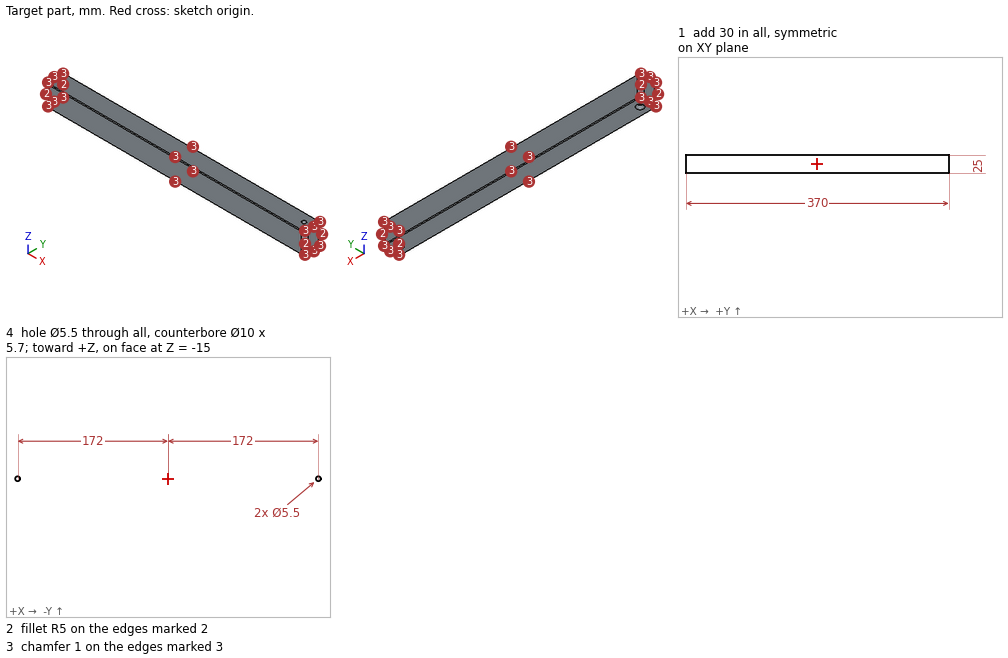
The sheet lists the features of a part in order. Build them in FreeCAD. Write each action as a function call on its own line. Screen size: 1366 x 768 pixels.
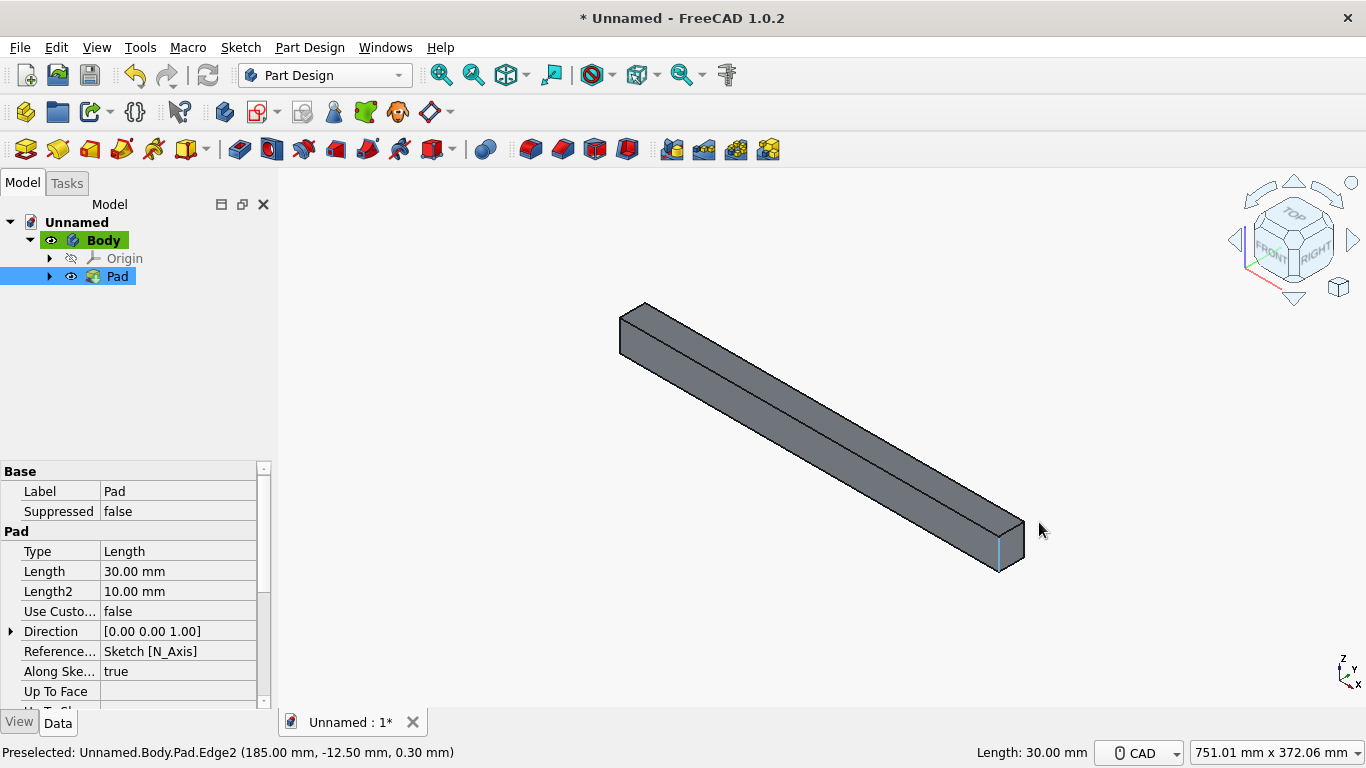
key(2)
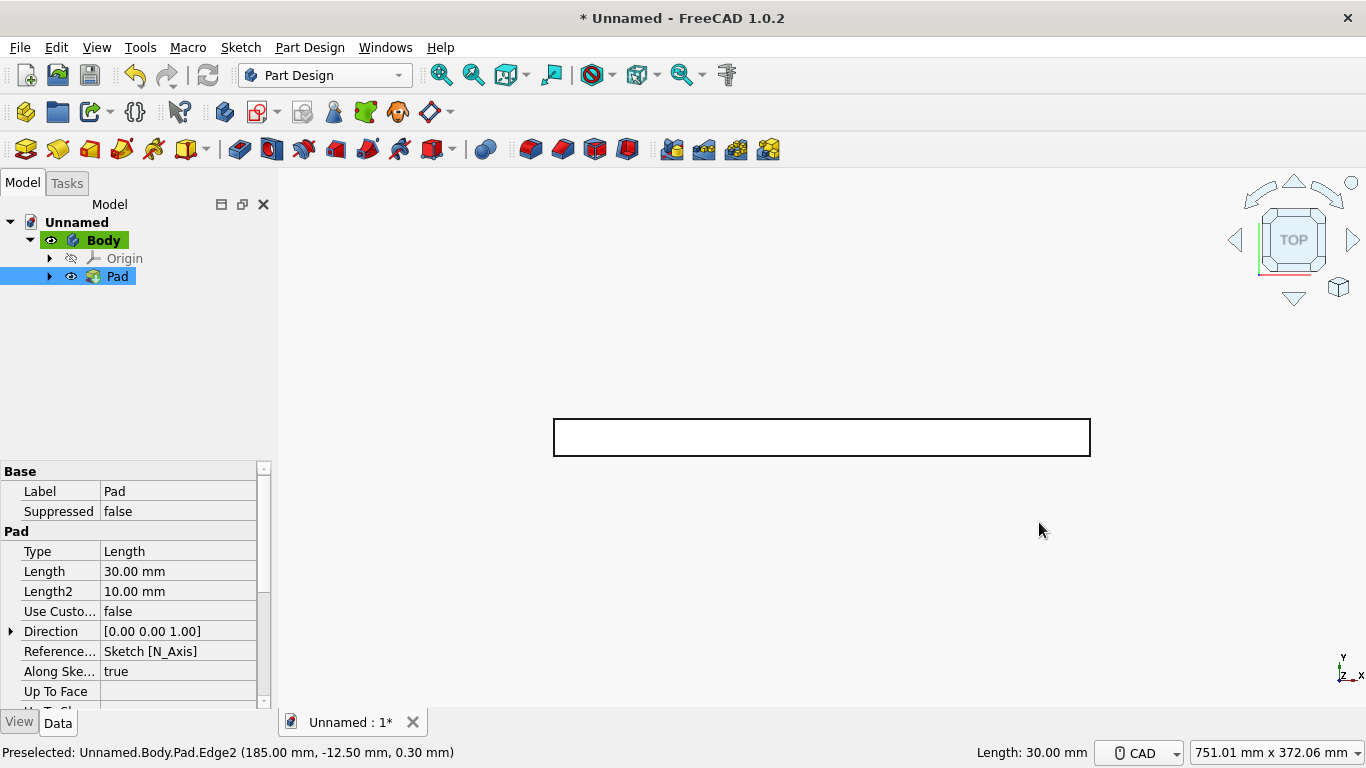
key(1)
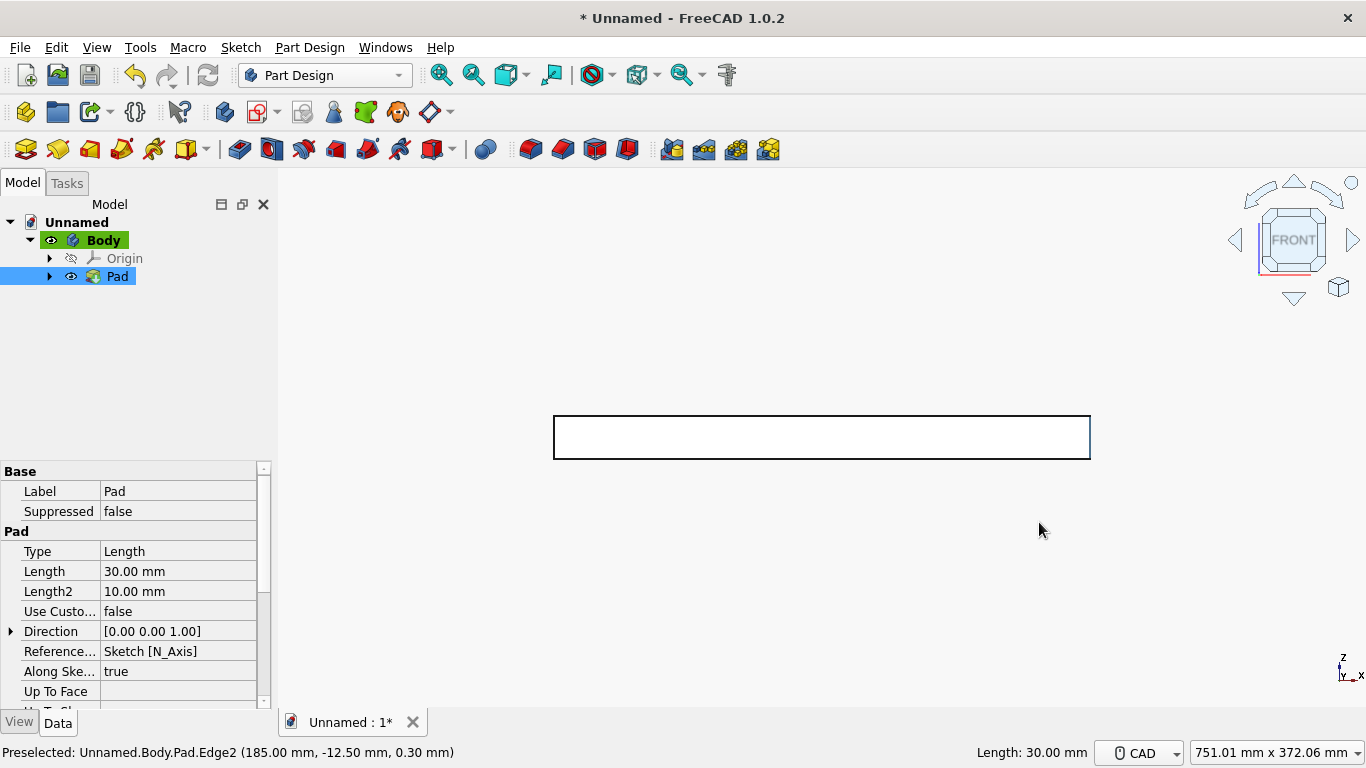
click(554, 436, ctrl)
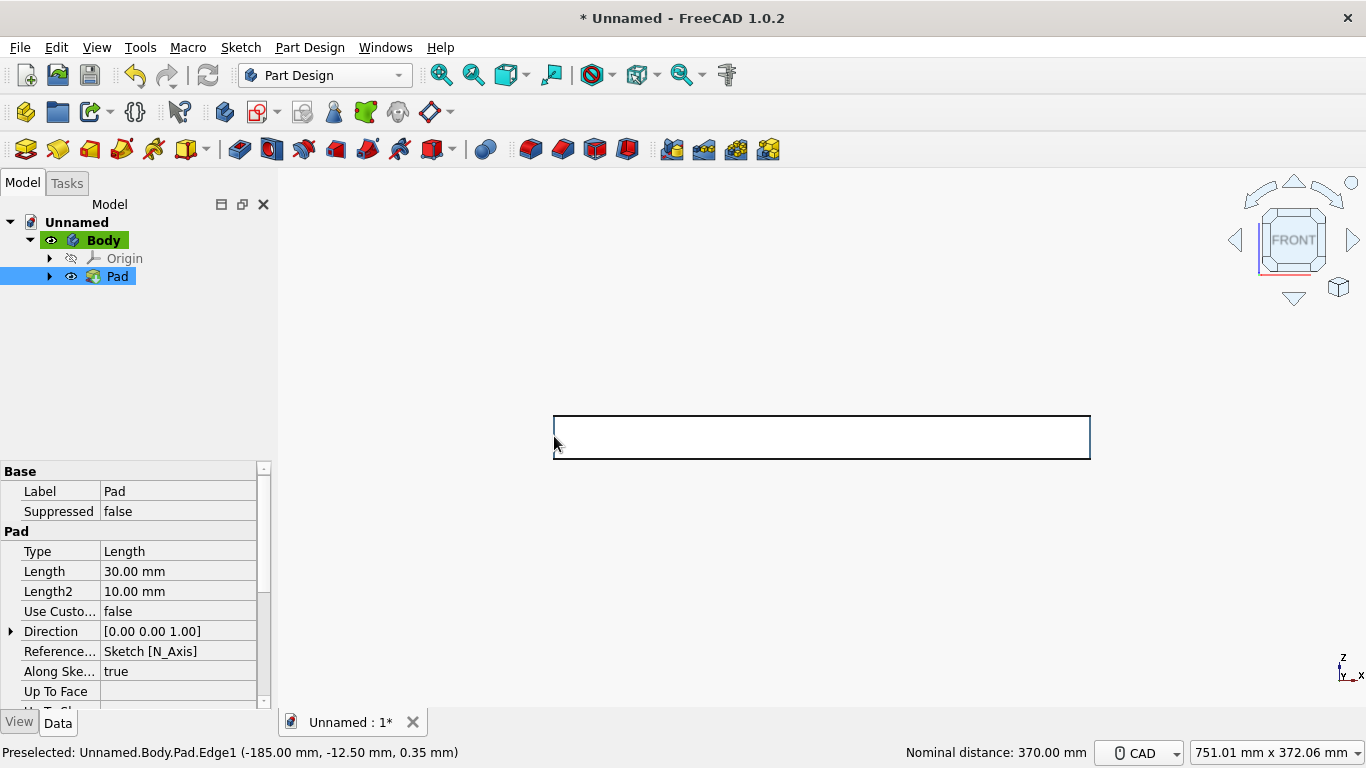
key(3)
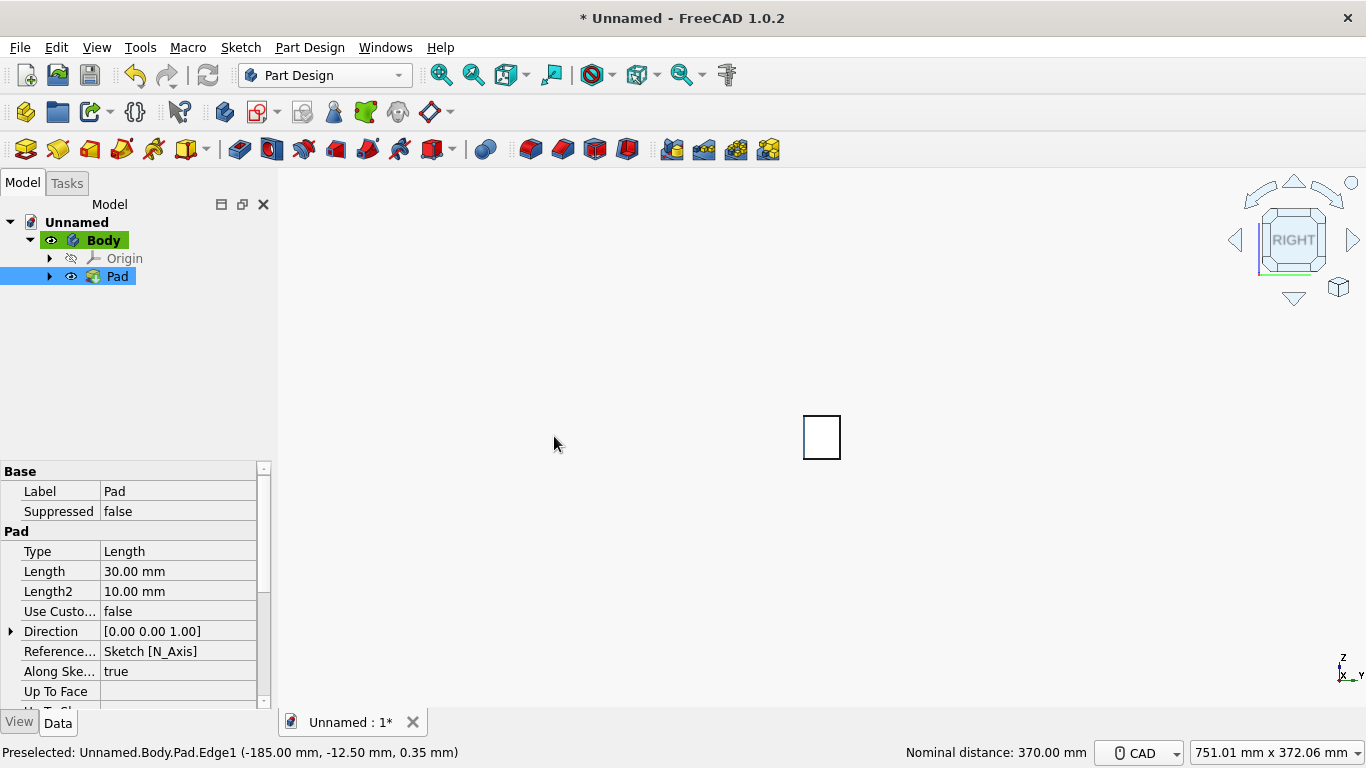
click(442, 76)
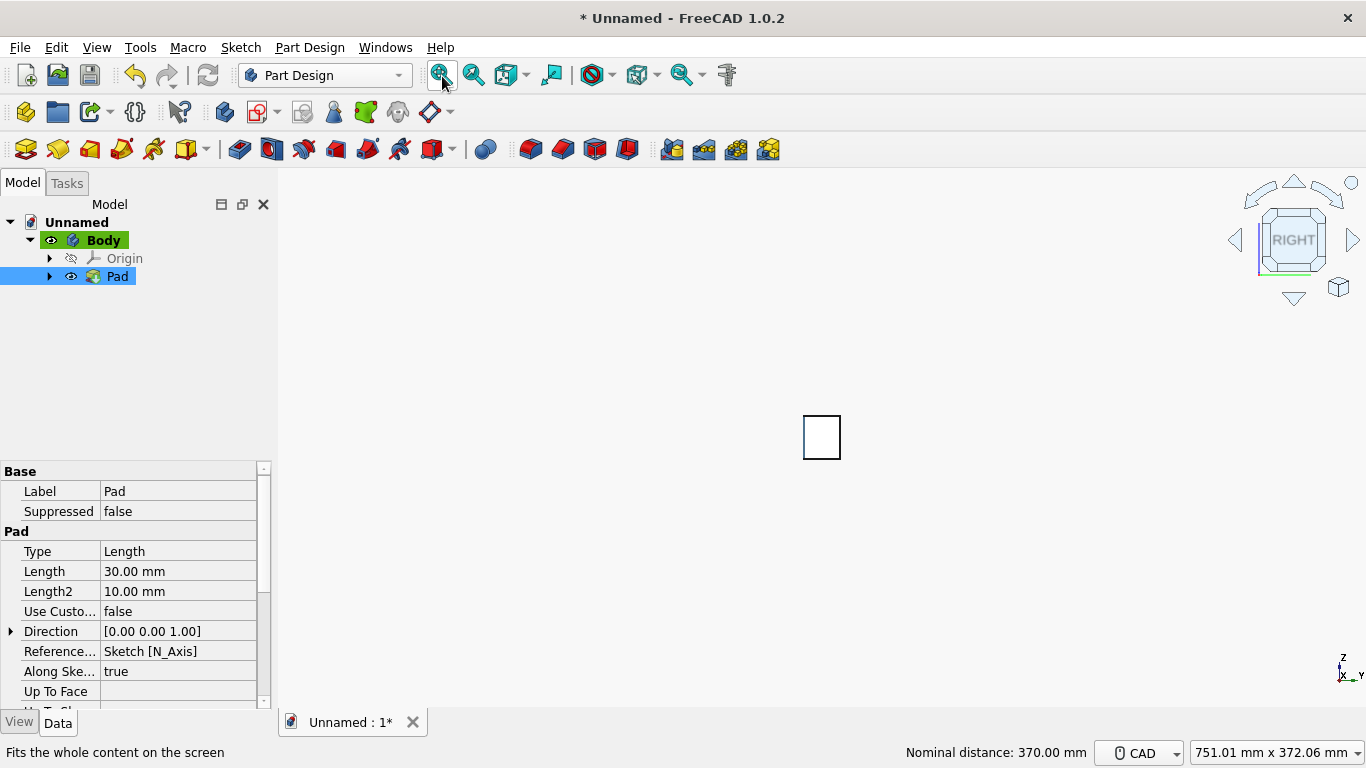
click(840, 436, ctrl)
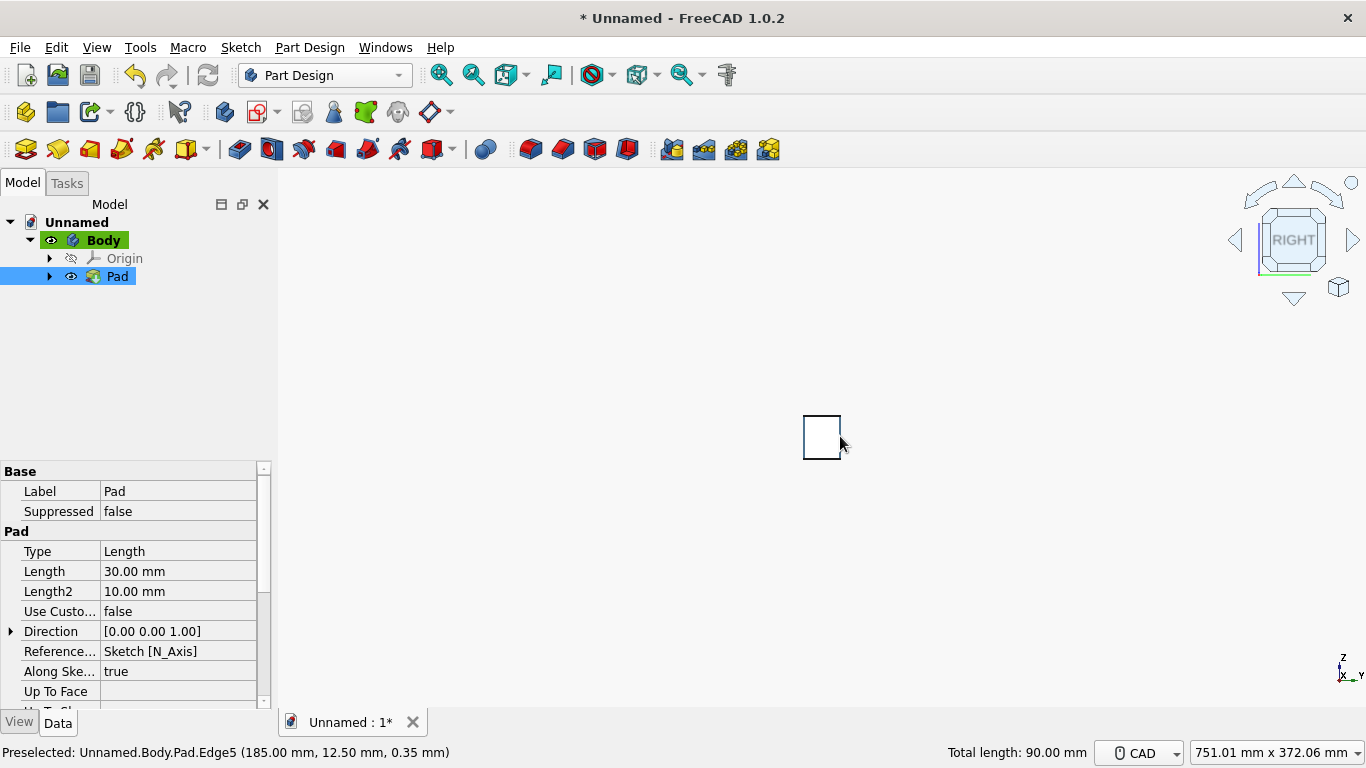
key(5)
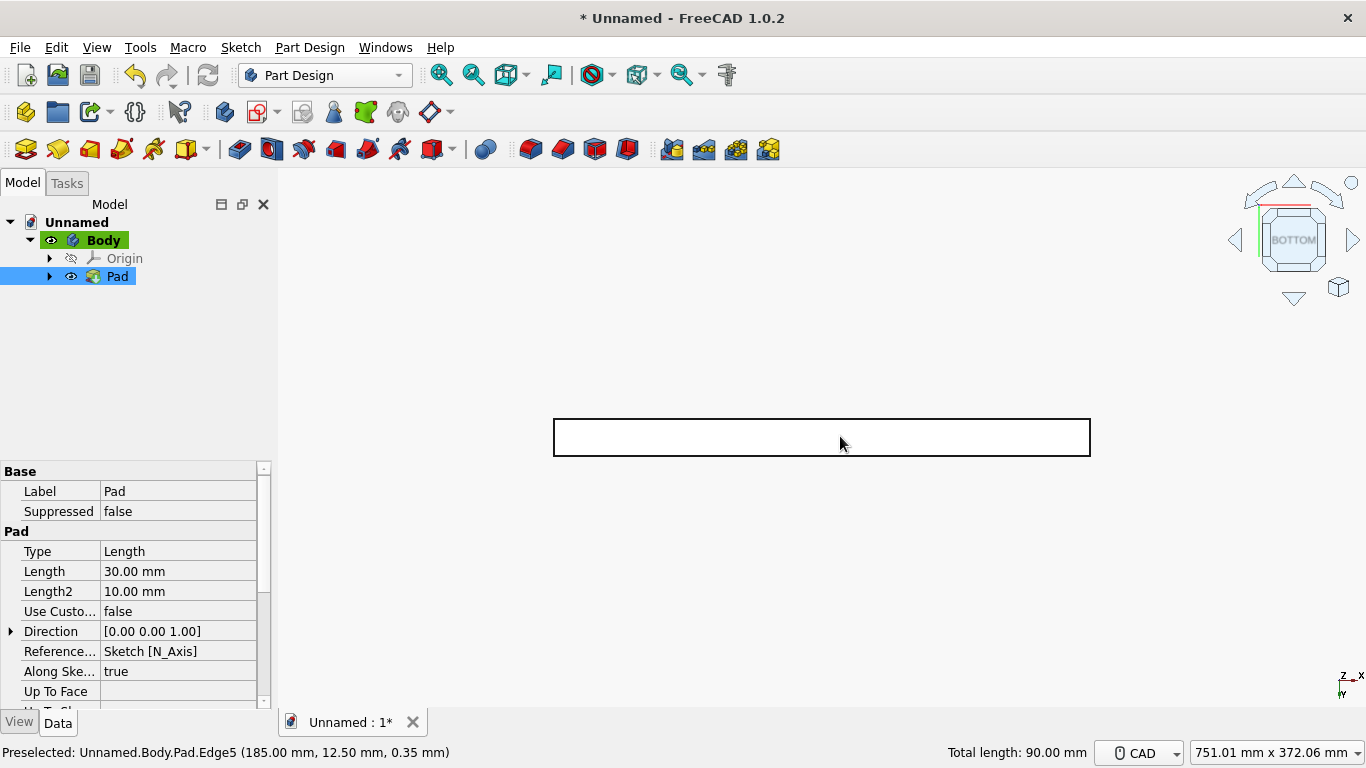
key(4)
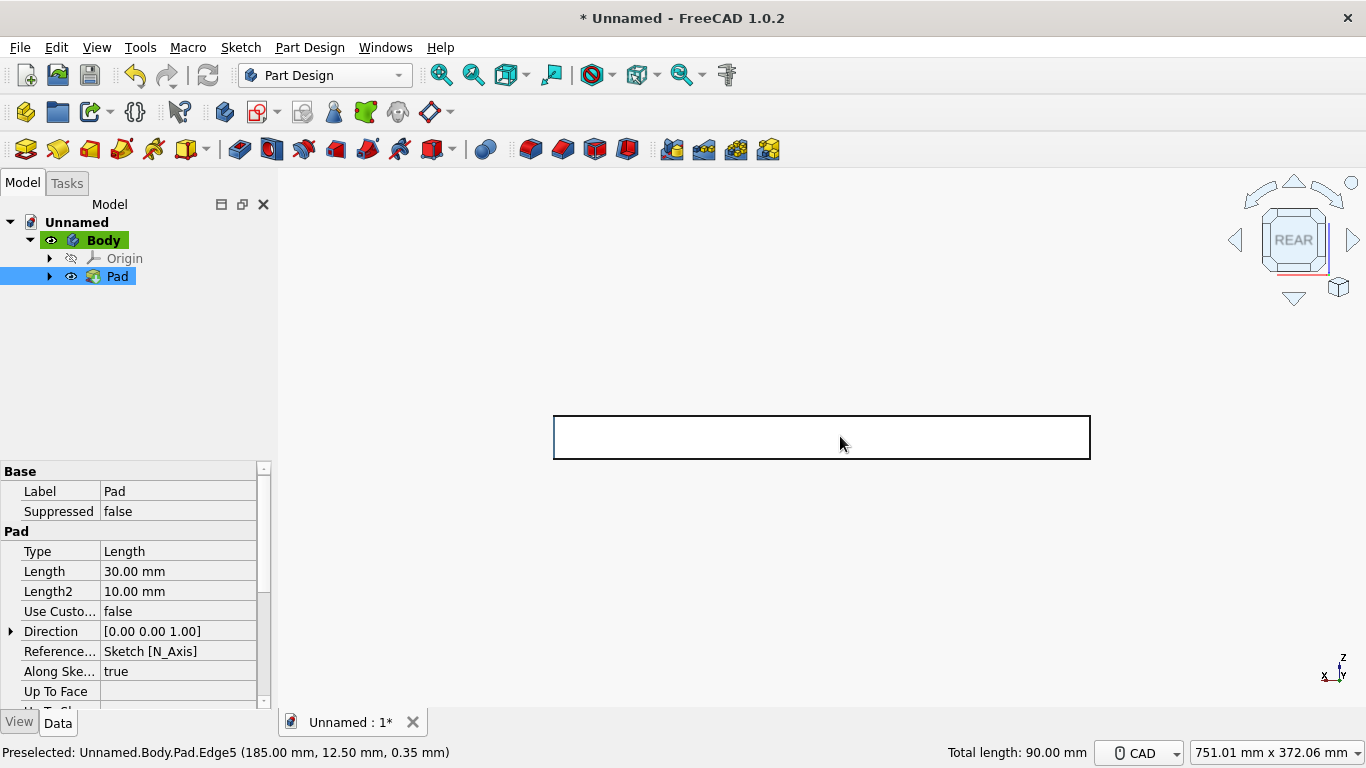
click(1090, 436, ctrl)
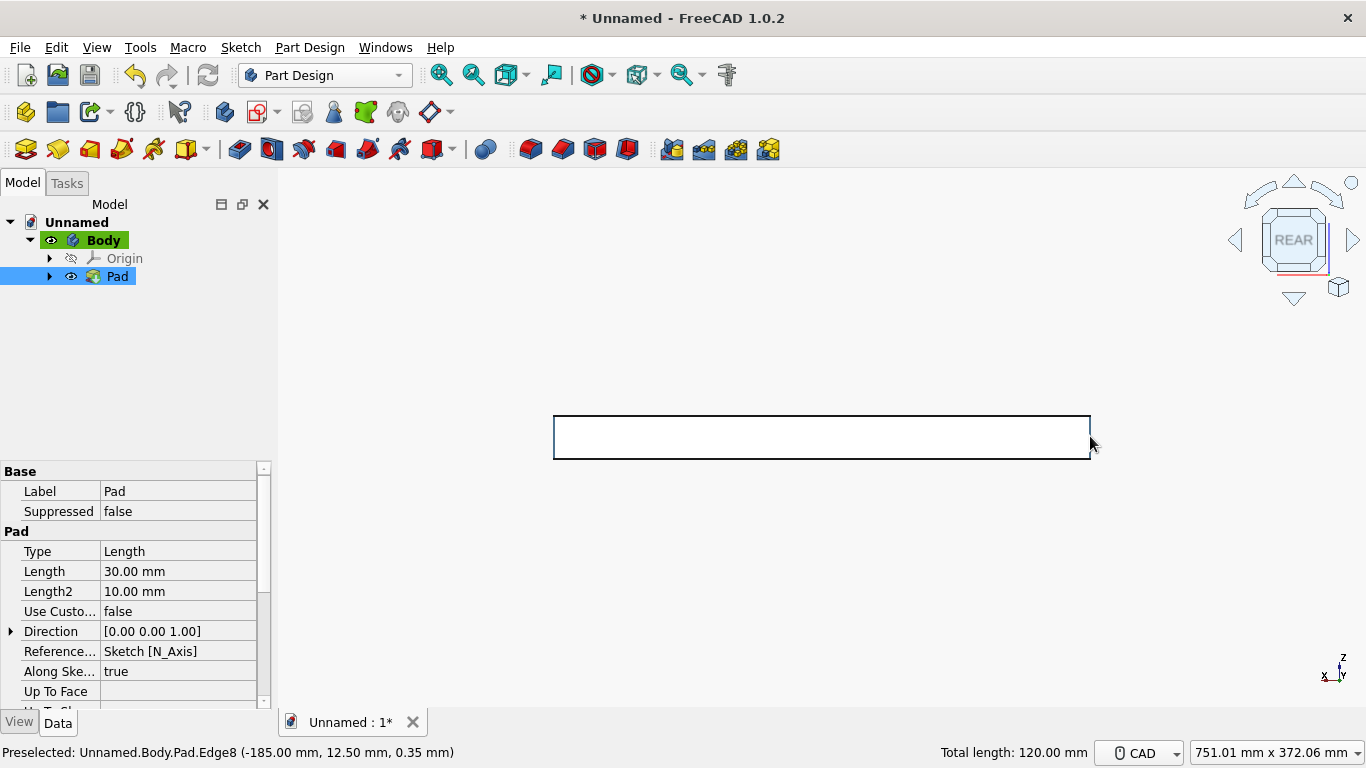
click(532, 150)